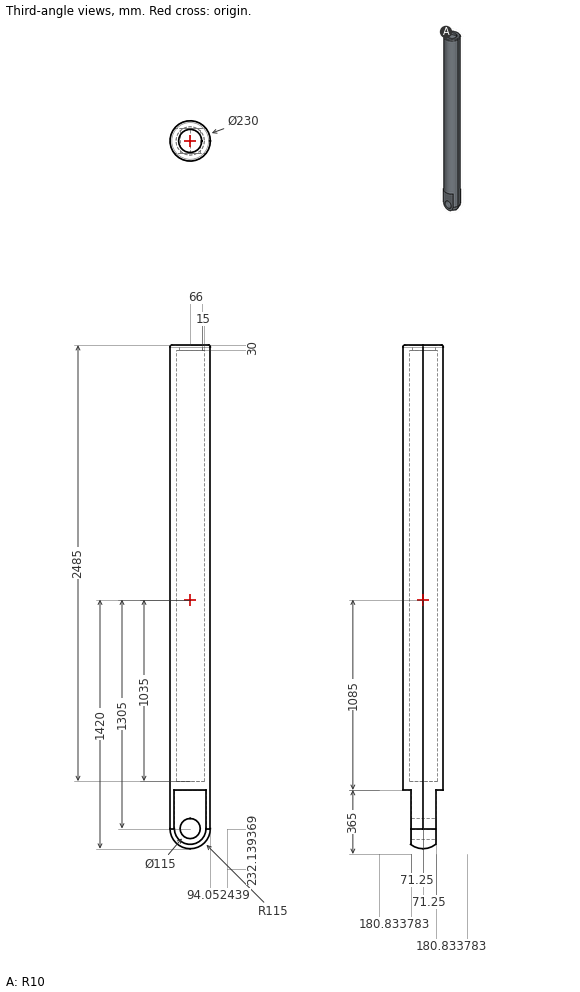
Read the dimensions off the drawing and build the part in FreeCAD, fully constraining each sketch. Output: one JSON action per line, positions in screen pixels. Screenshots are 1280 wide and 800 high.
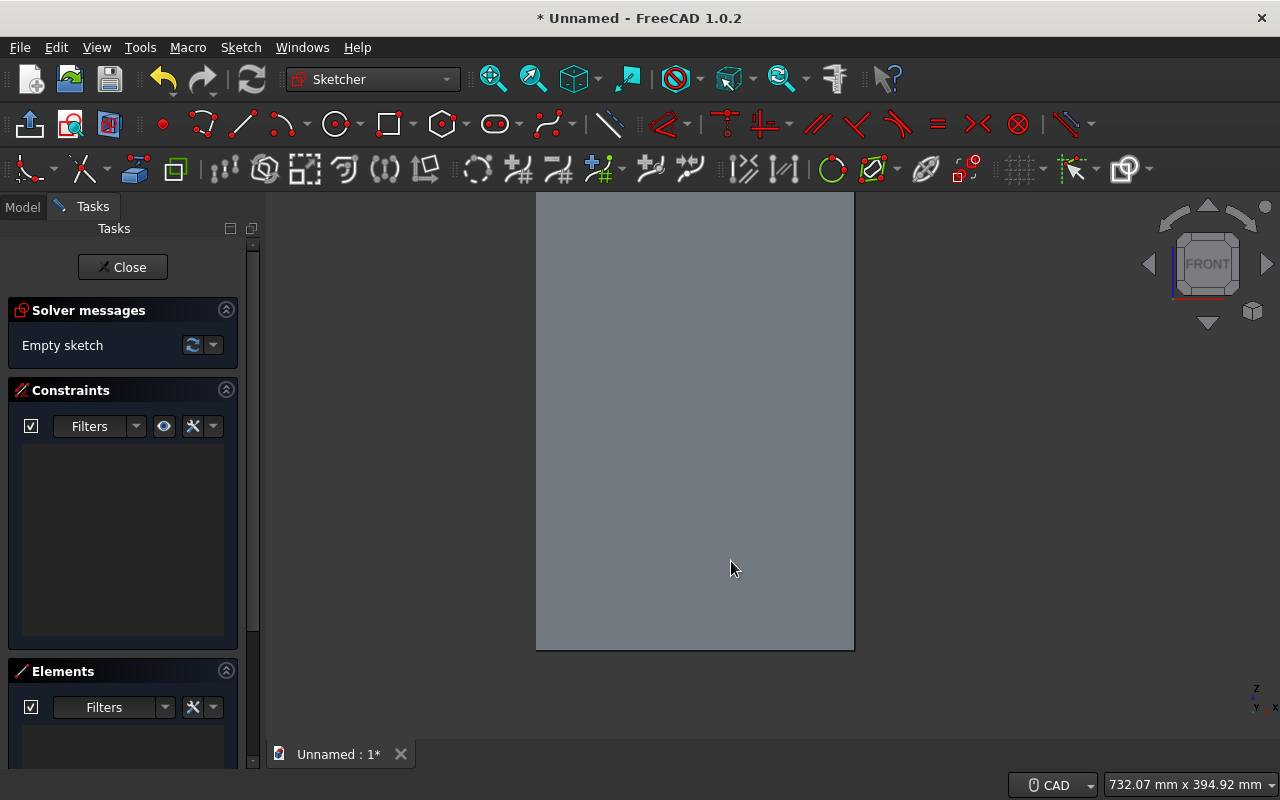
{"action": "scroll", "coordinate": [688, 438], "scroll_direction": "up", "scroll_amount": 4}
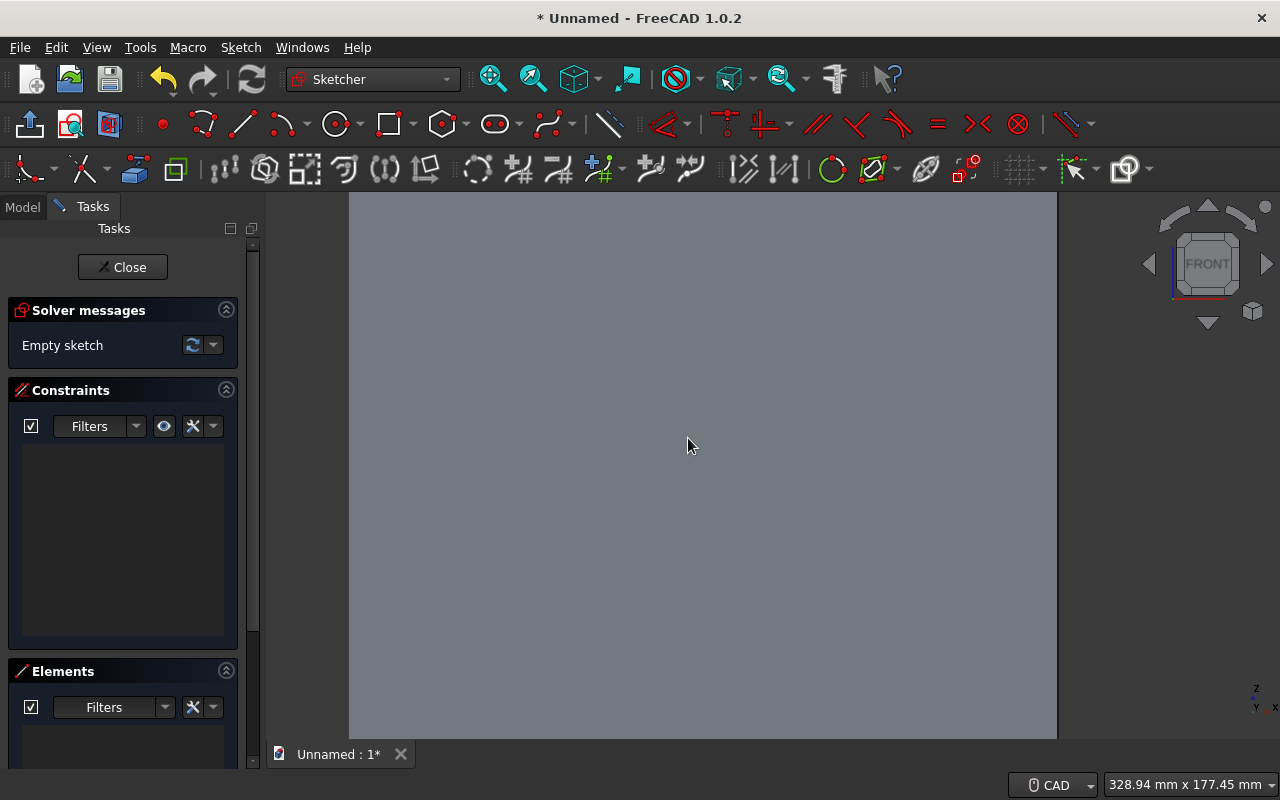
{"action": "key", "text": "g c"}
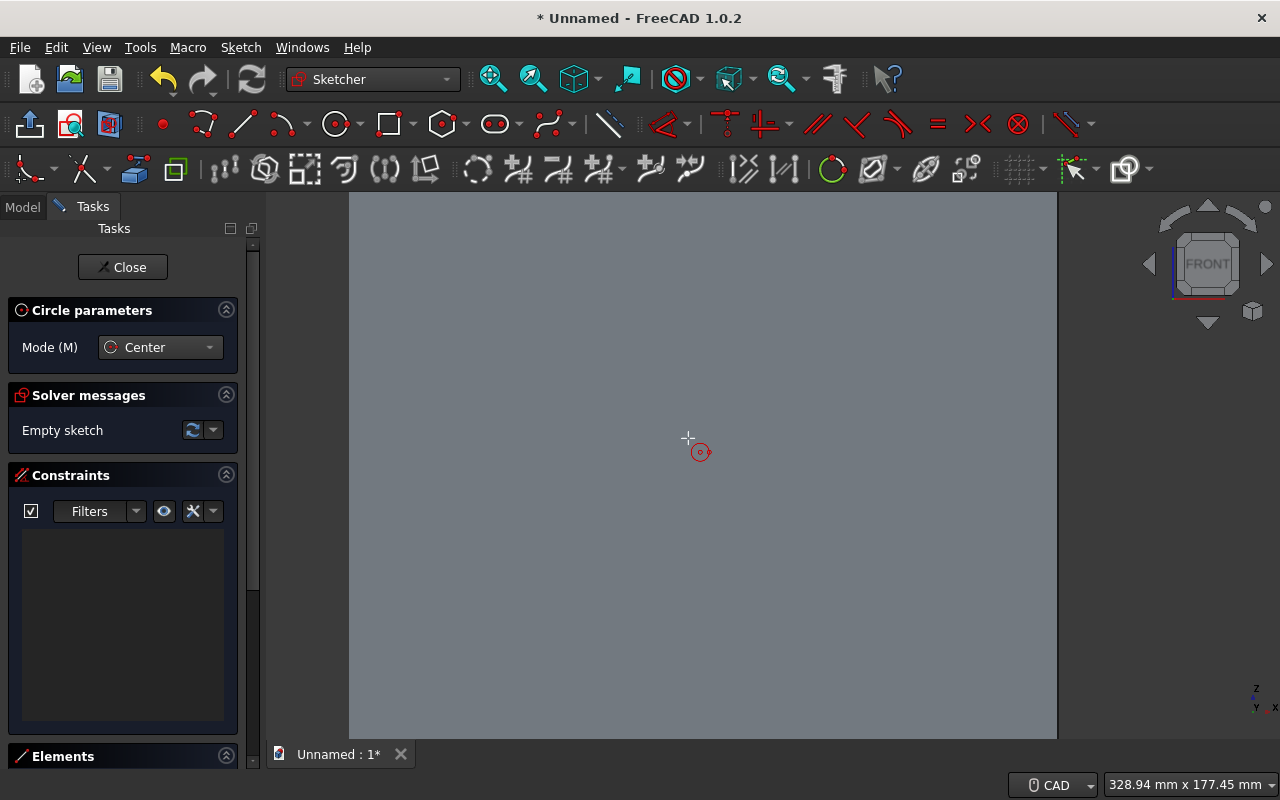
{"action": "left_click", "coordinate": [704, 465]}
{"action": "mouse_move", "coordinate": [829, 339]}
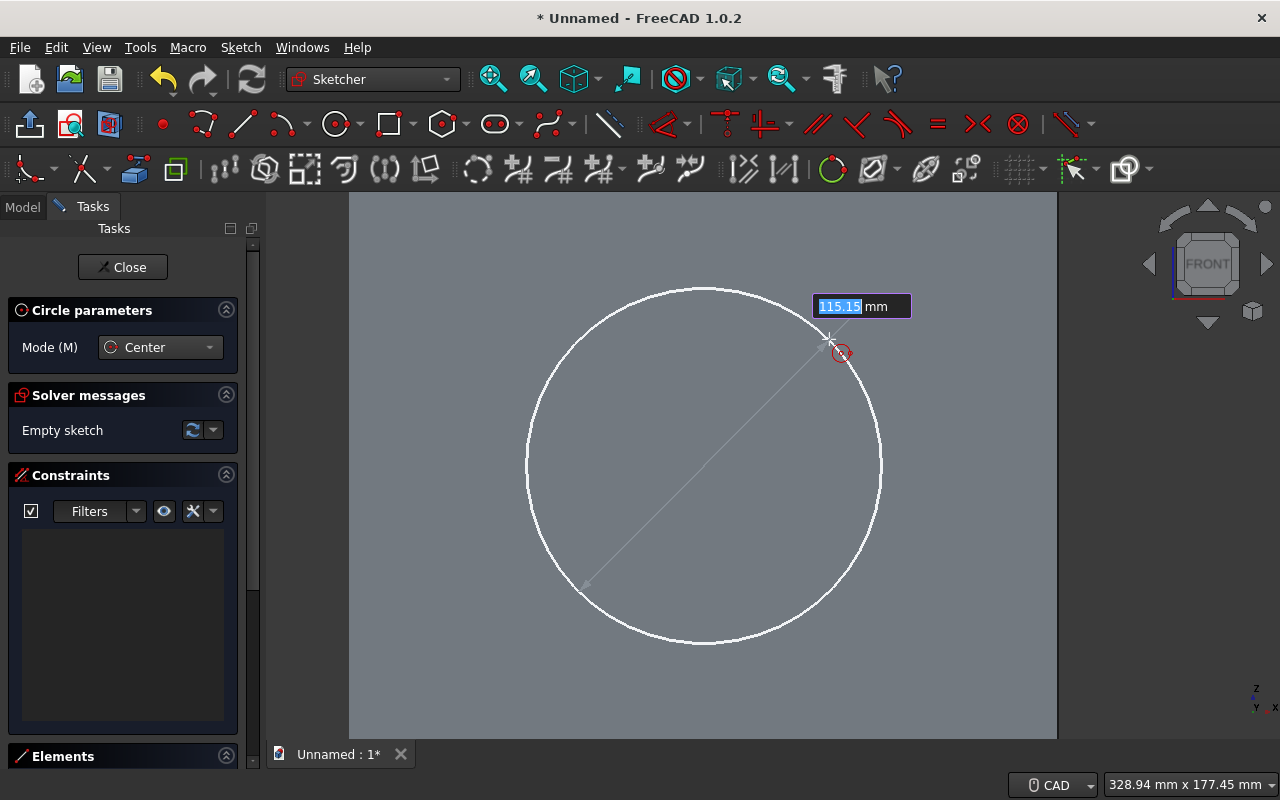
{"action": "type", "text": "115"}
{"action": "key", "text": "Return"}
{"action": "key", "text": "Escape"}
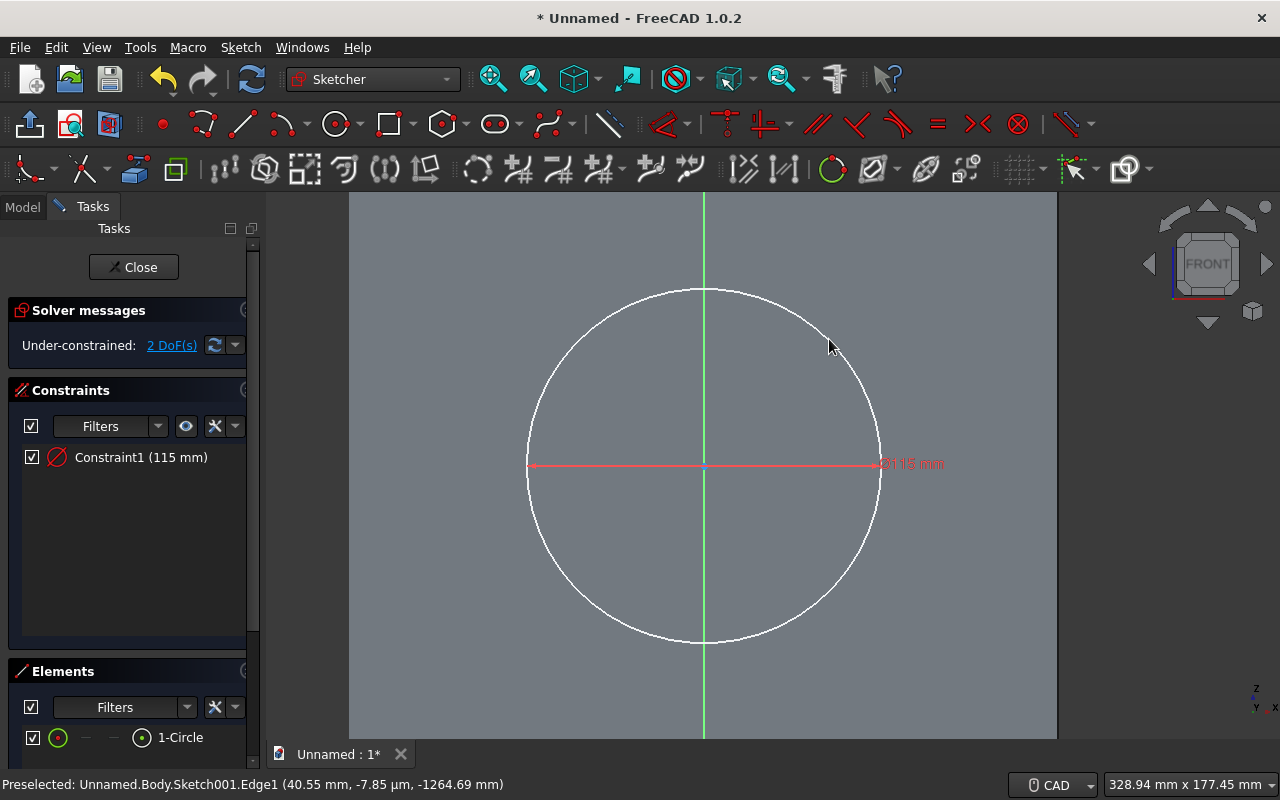
{"action": "left_click", "coordinate": [704, 466]}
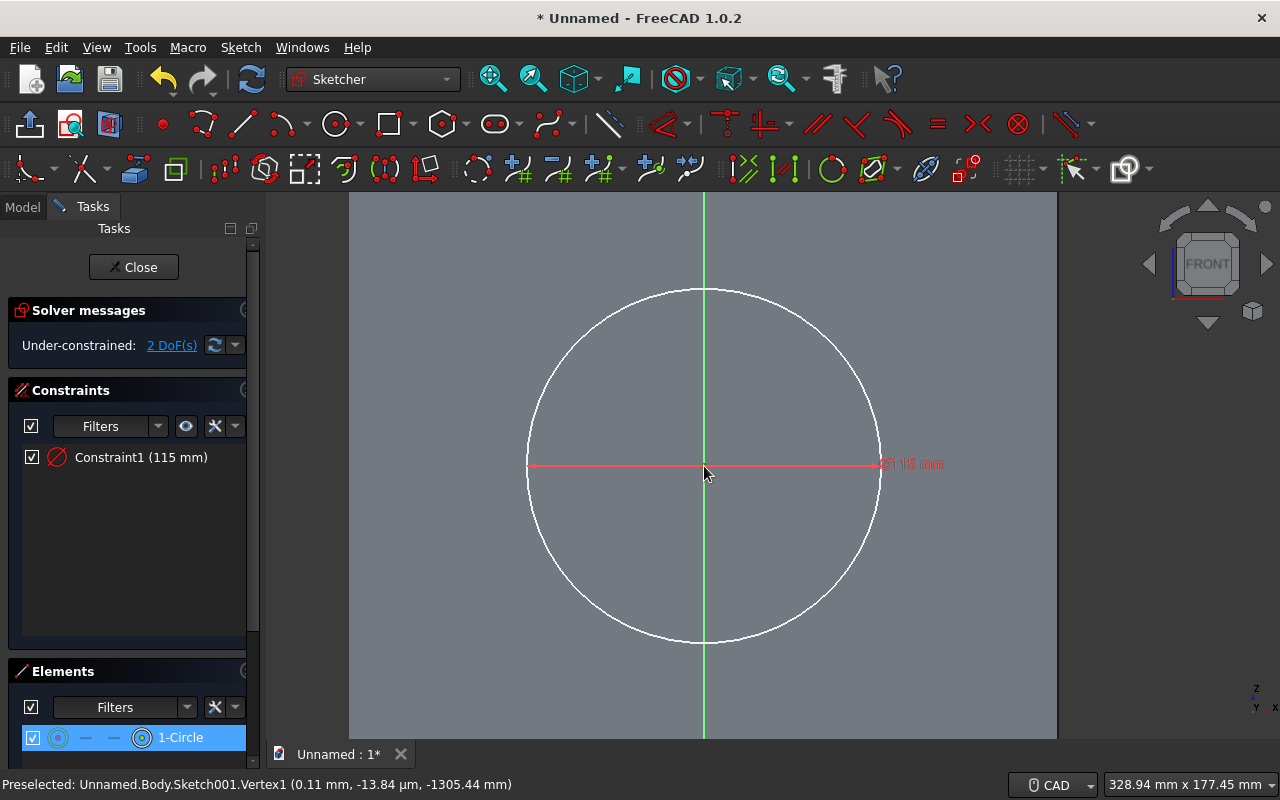
{"action": "left_click", "coordinate": [704, 676]}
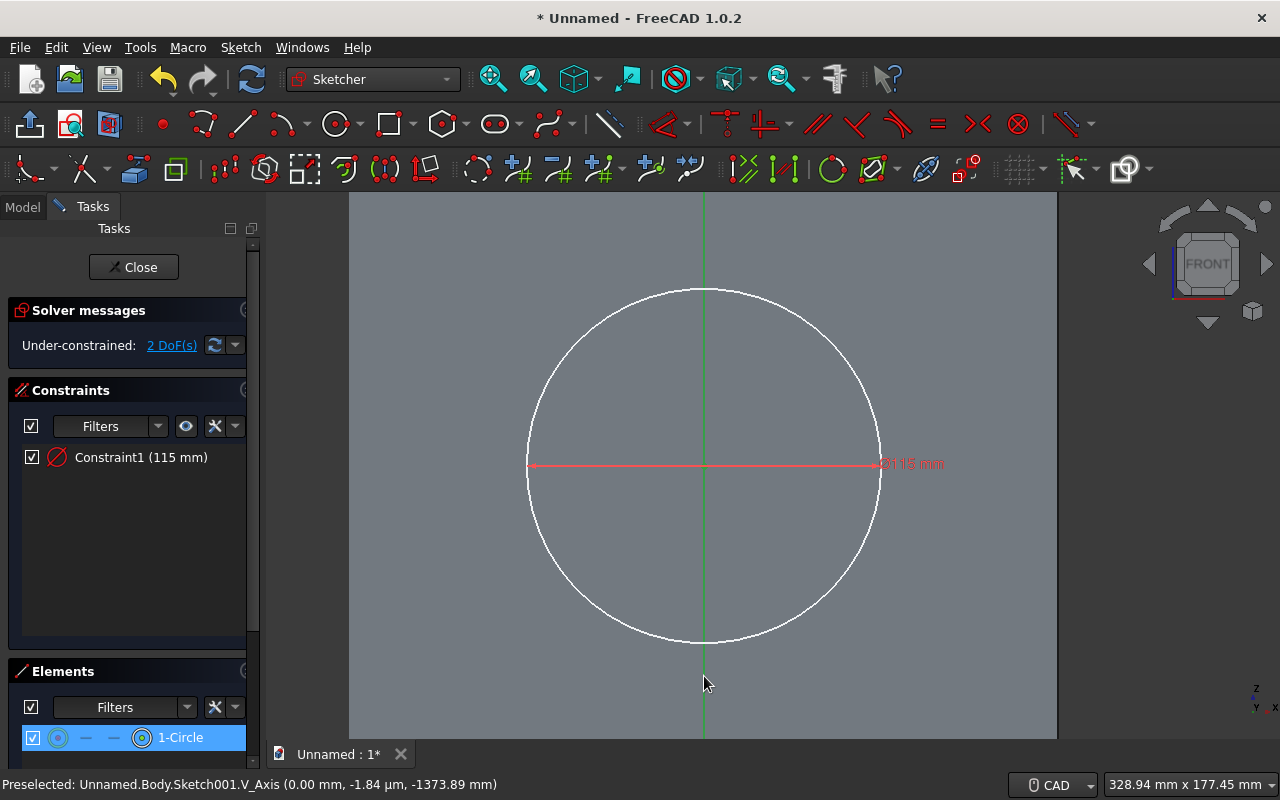
{"action": "left_click", "coordinate": [726, 124]}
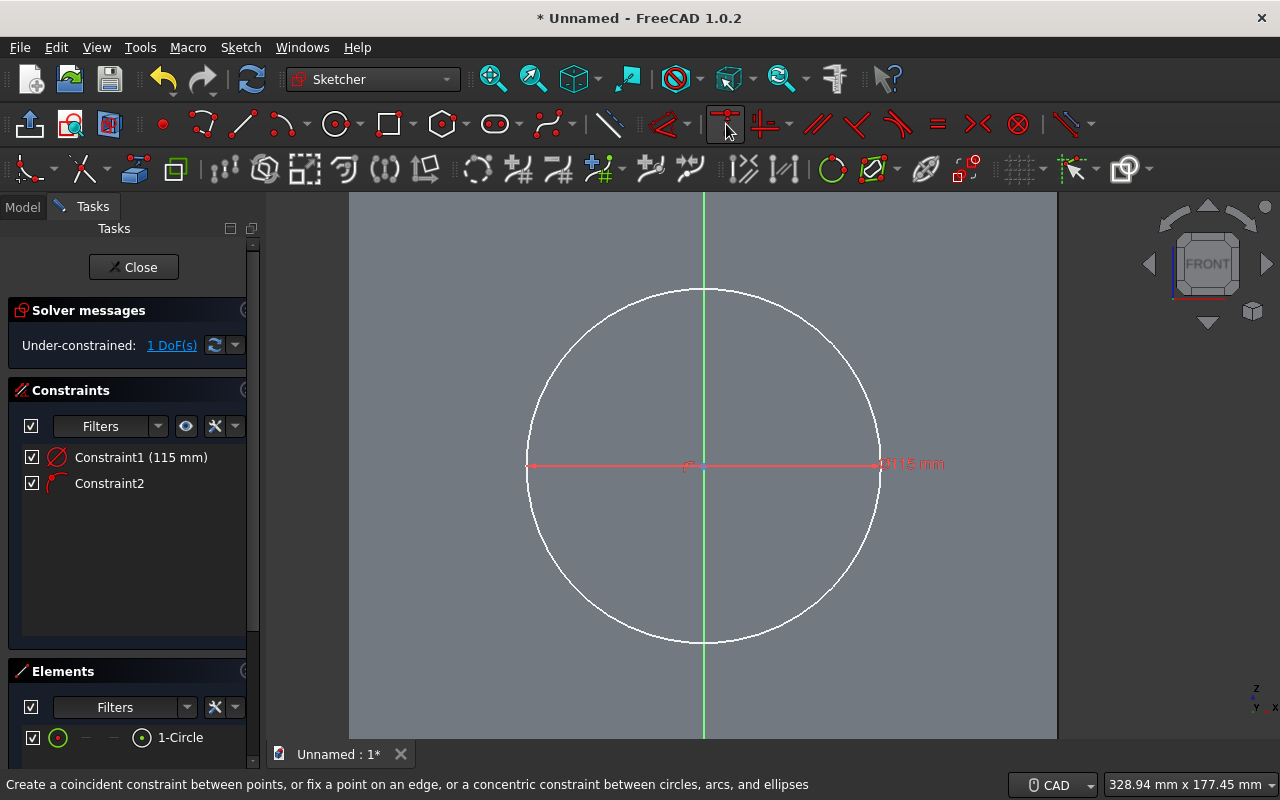
{"action": "key", "text": "d"}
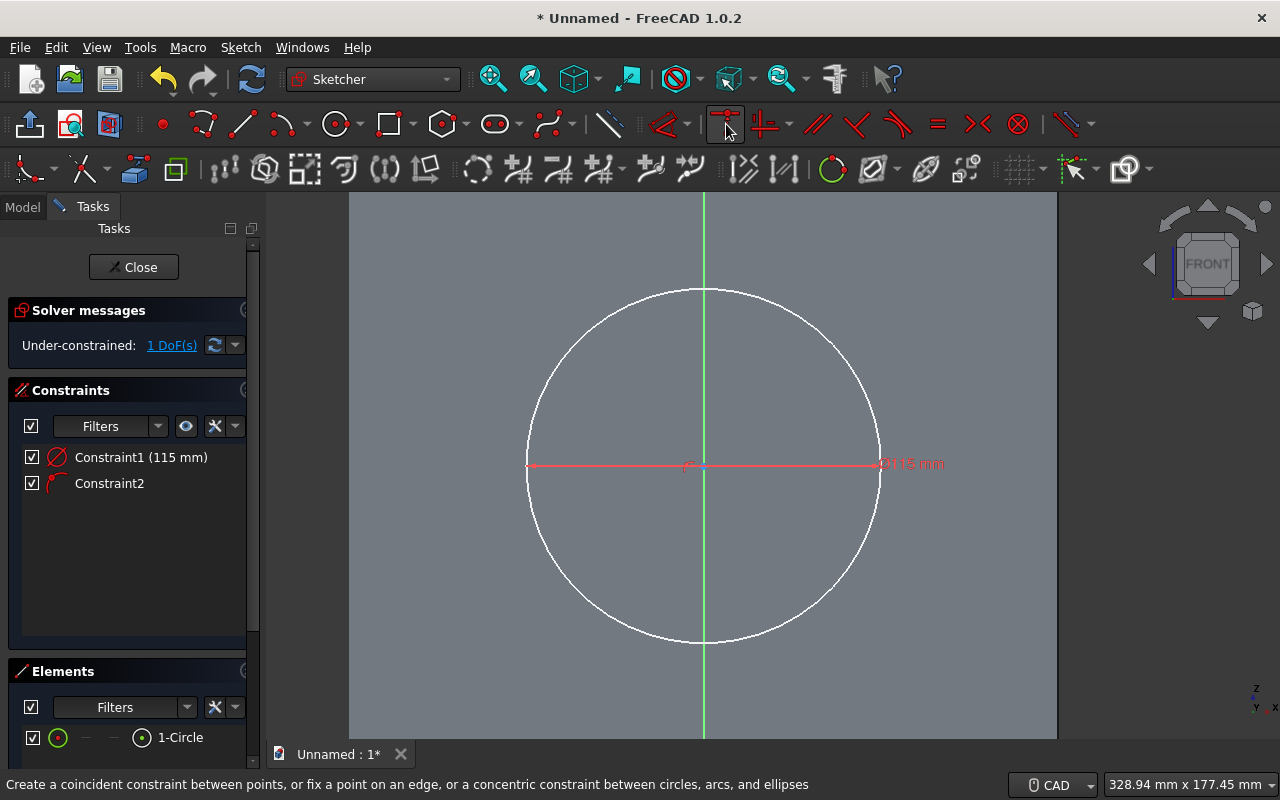
{"action": "left_click", "coordinate": [704, 466]}
{"action": "left_click", "coordinate": [738, 343]}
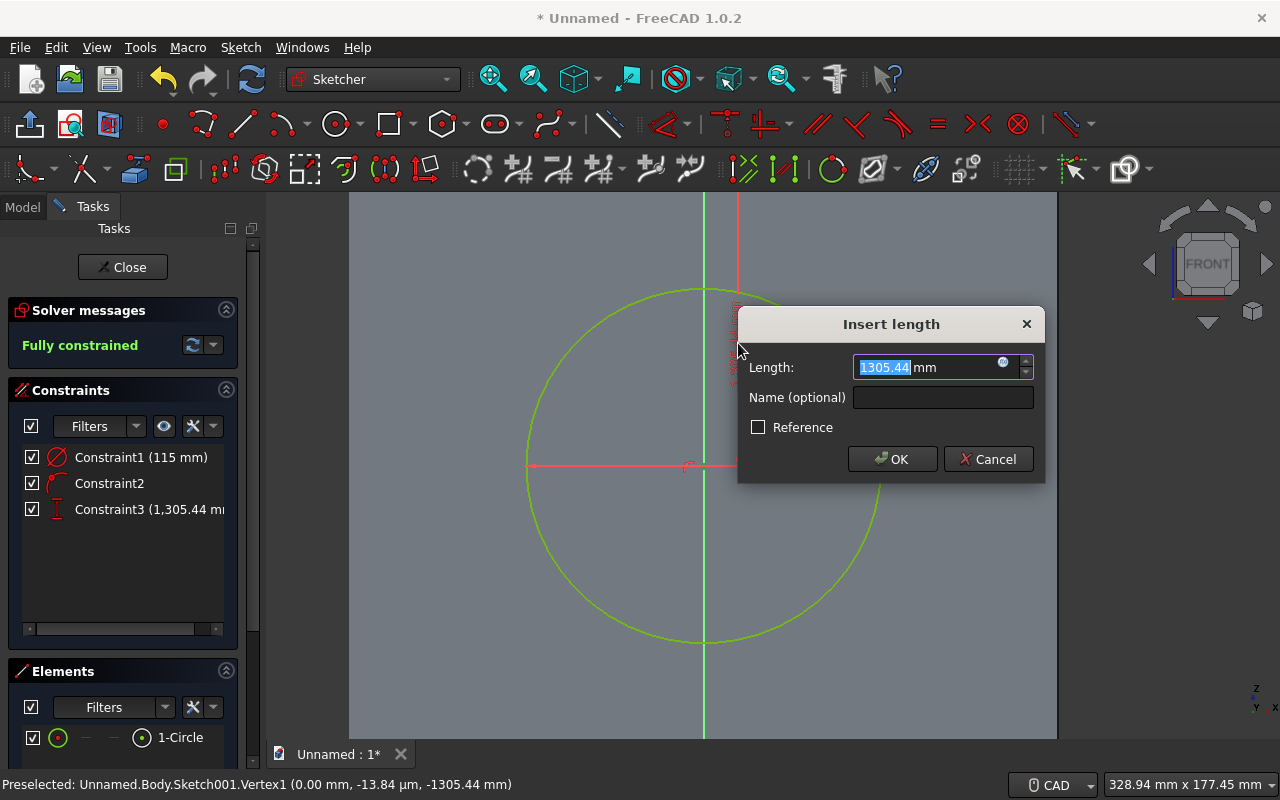
{"action": "type", "text": "1305"}
{"action": "key", "text": "Return"}
{"action": "key", "text": "Escape"}